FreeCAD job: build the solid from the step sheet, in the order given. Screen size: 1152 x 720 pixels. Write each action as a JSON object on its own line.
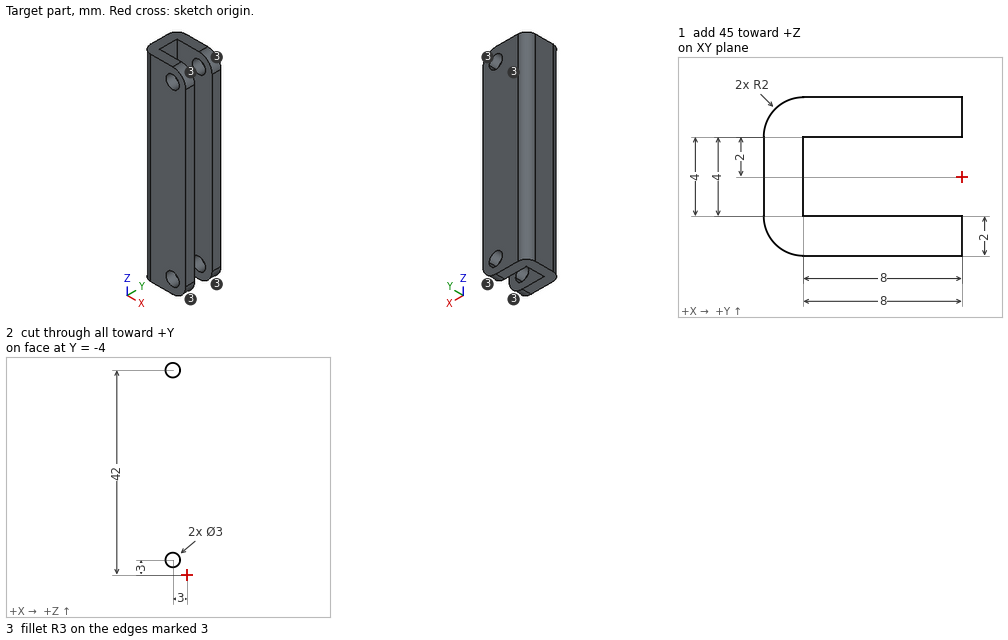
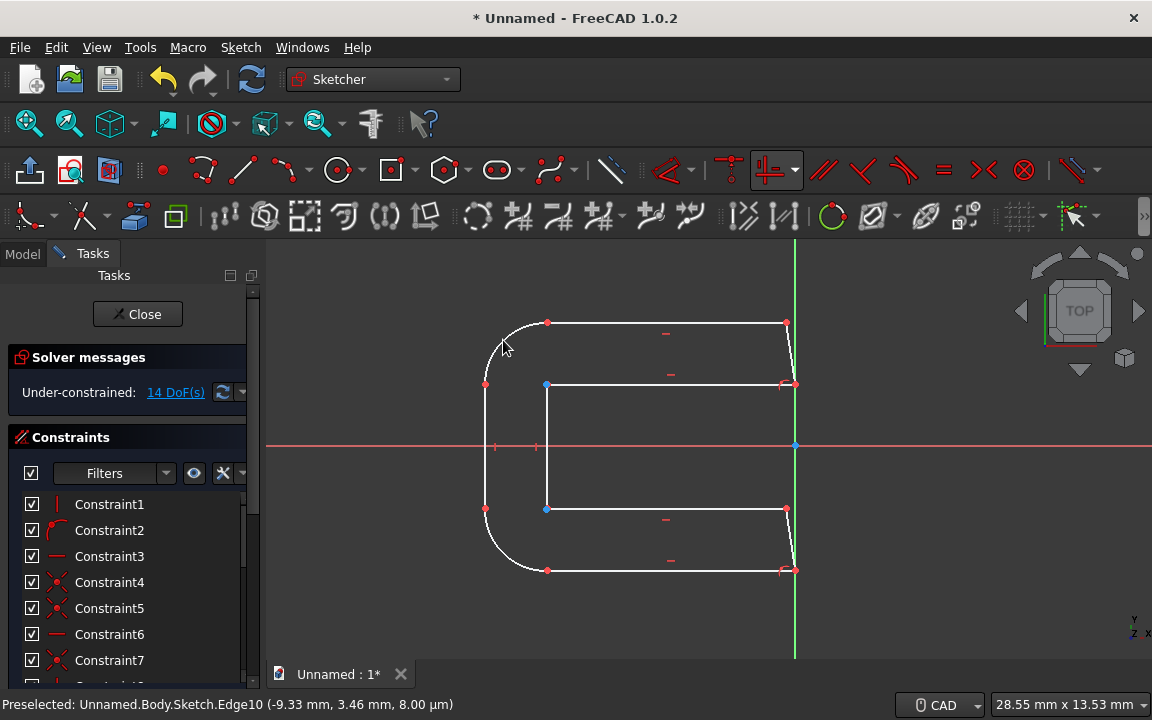
{"action": "left_click", "coordinate": [485, 422]}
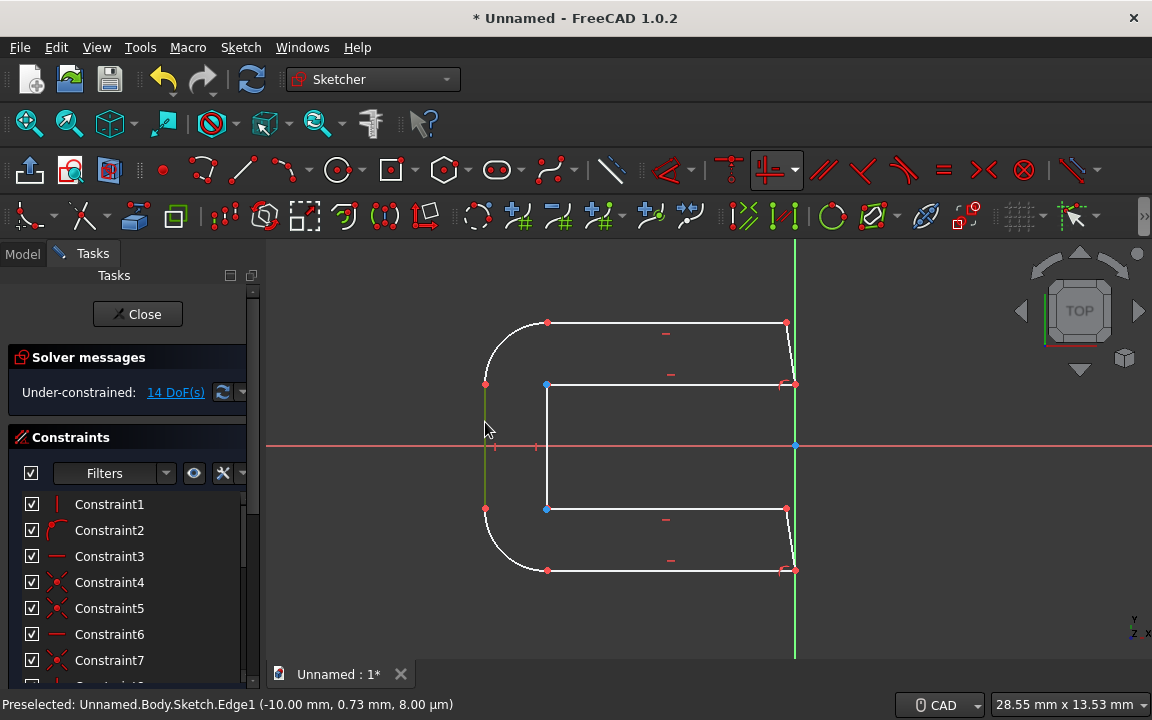
{"action": "left_click", "coordinate": [492, 537]}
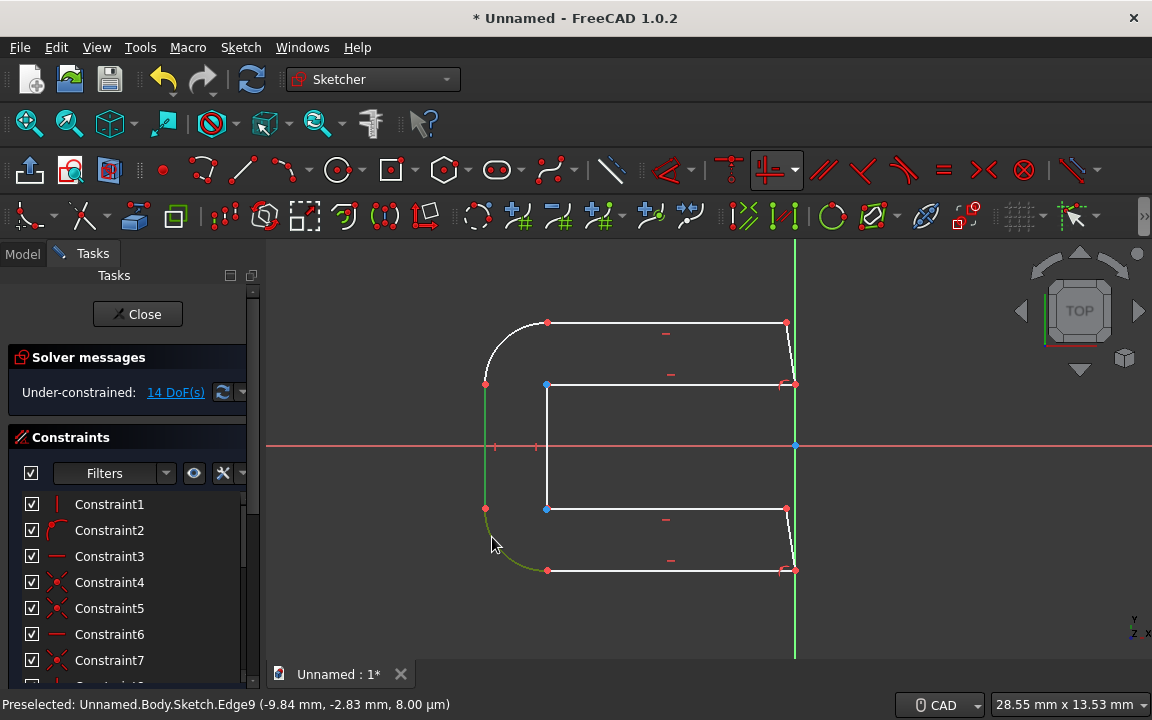
{"action": "left_click", "coordinate": [904, 170]}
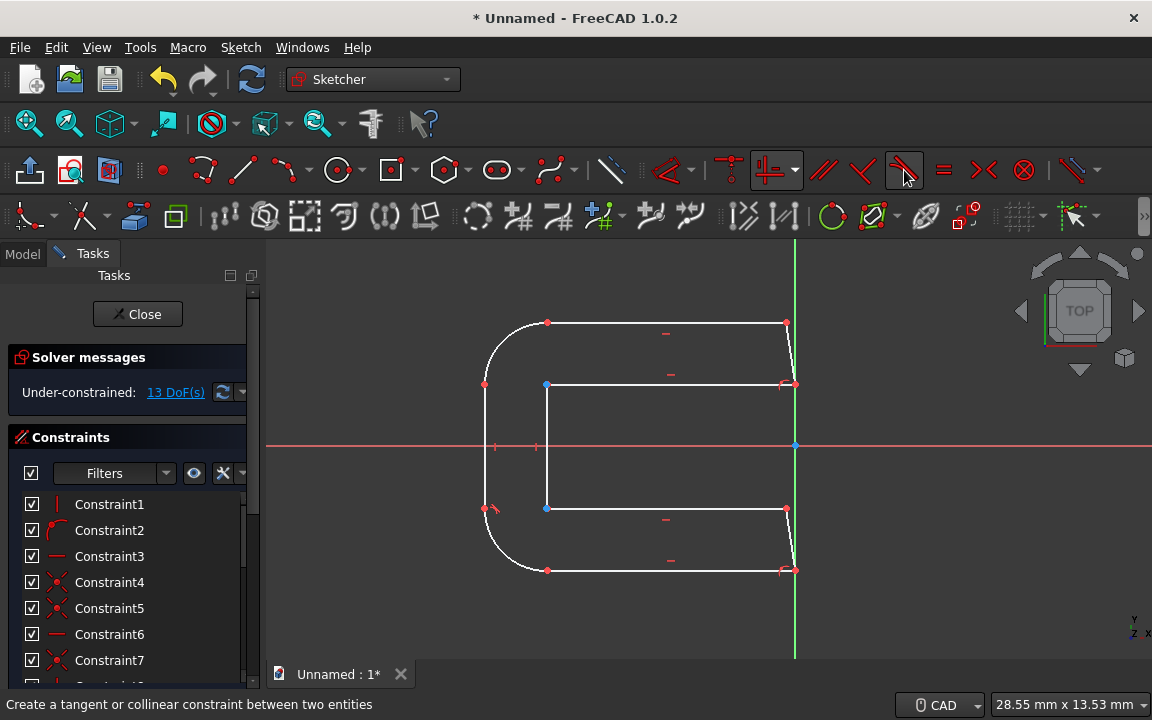
{"action": "left_click", "coordinate": [485, 422]}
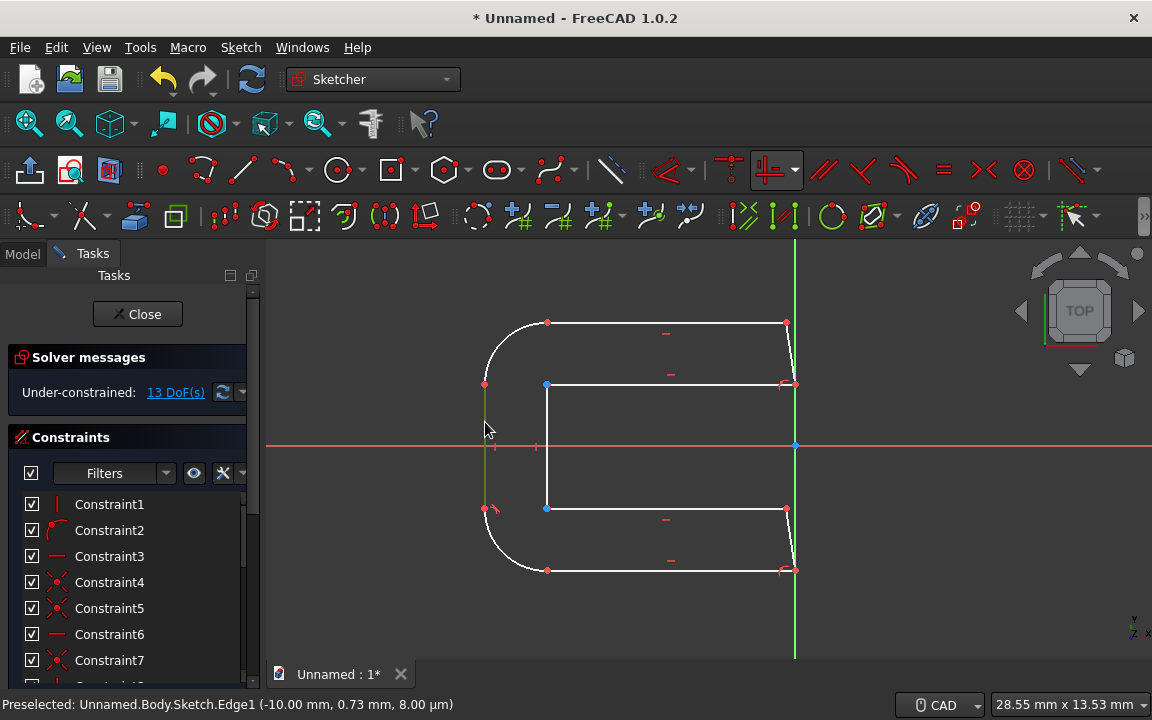
{"action": "left_click", "coordinate": [519, 330]}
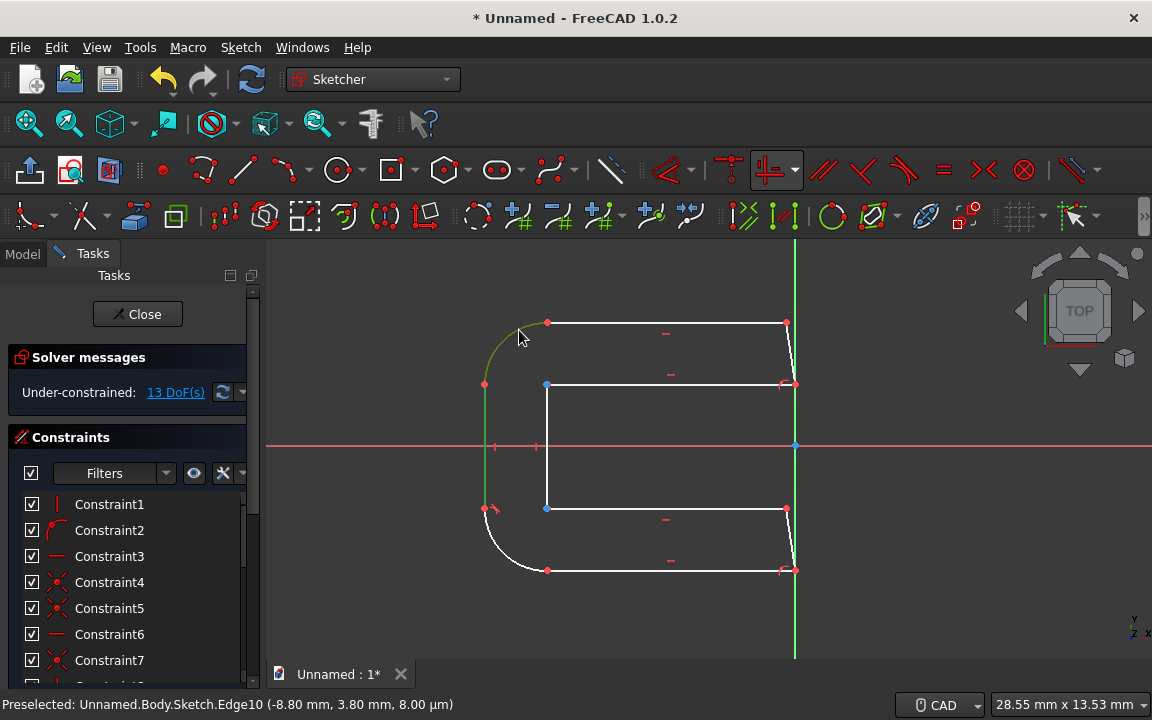
{"action": "left_click", "coordinate": [904, 170]}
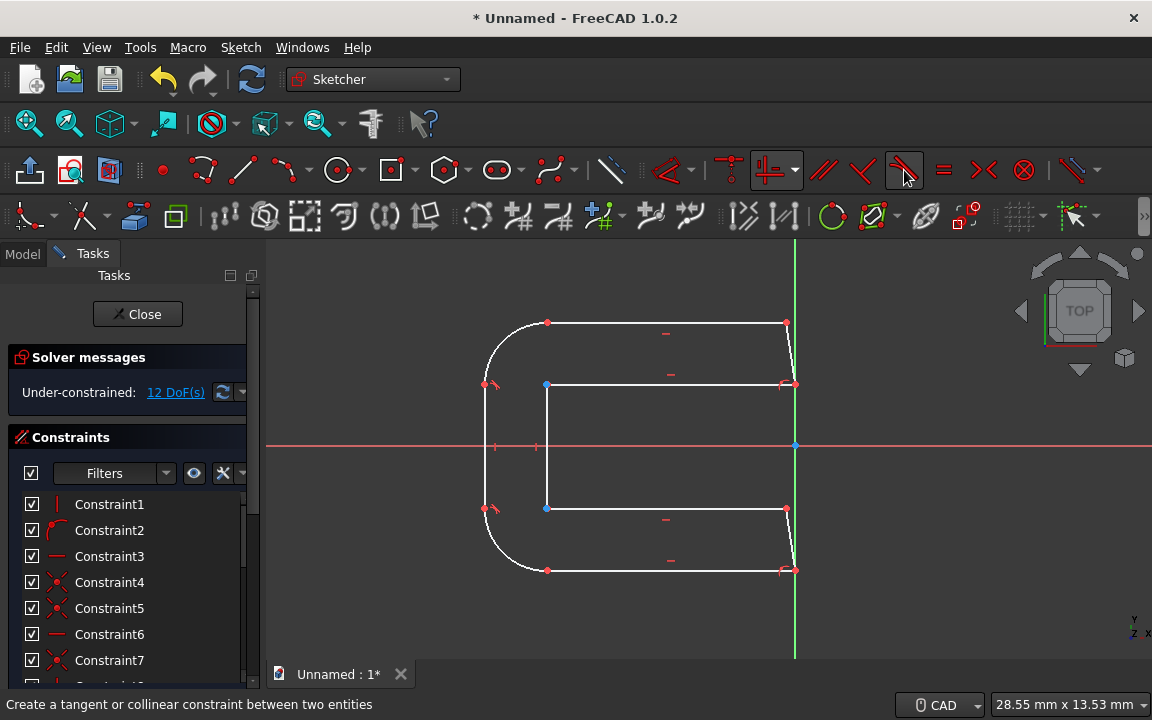
{"action": "left_click", "coordinate": [622, 571]}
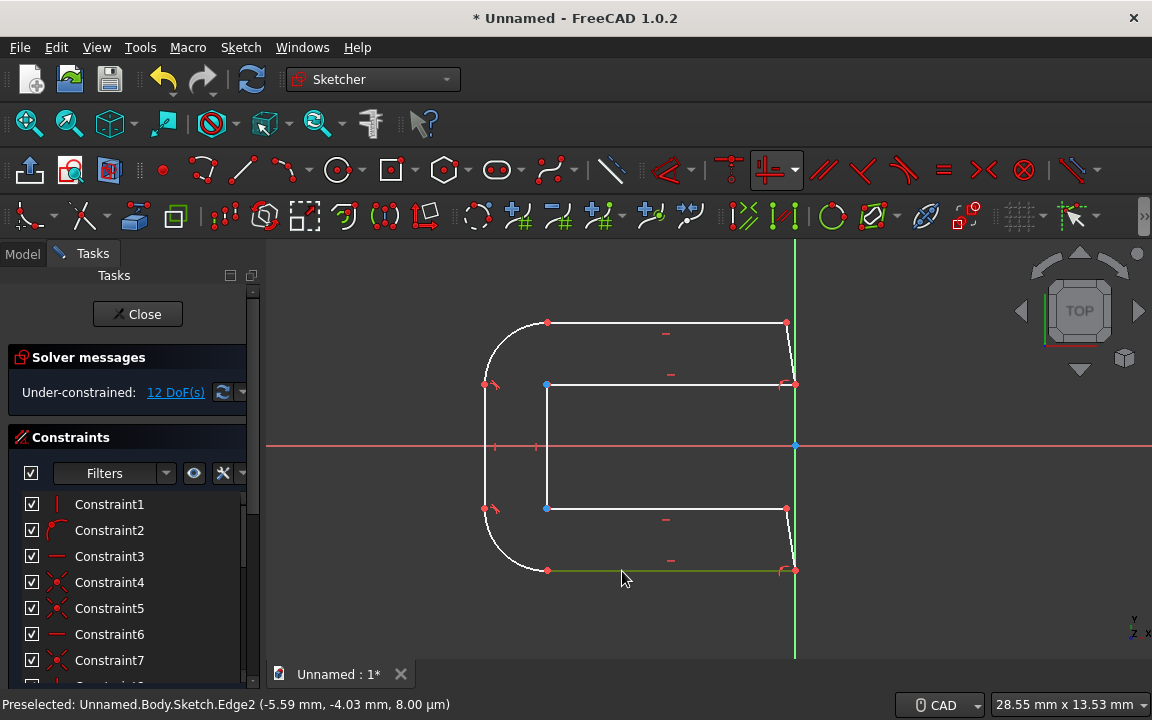
{"action": "left_click", "coordinate": [492, 537]}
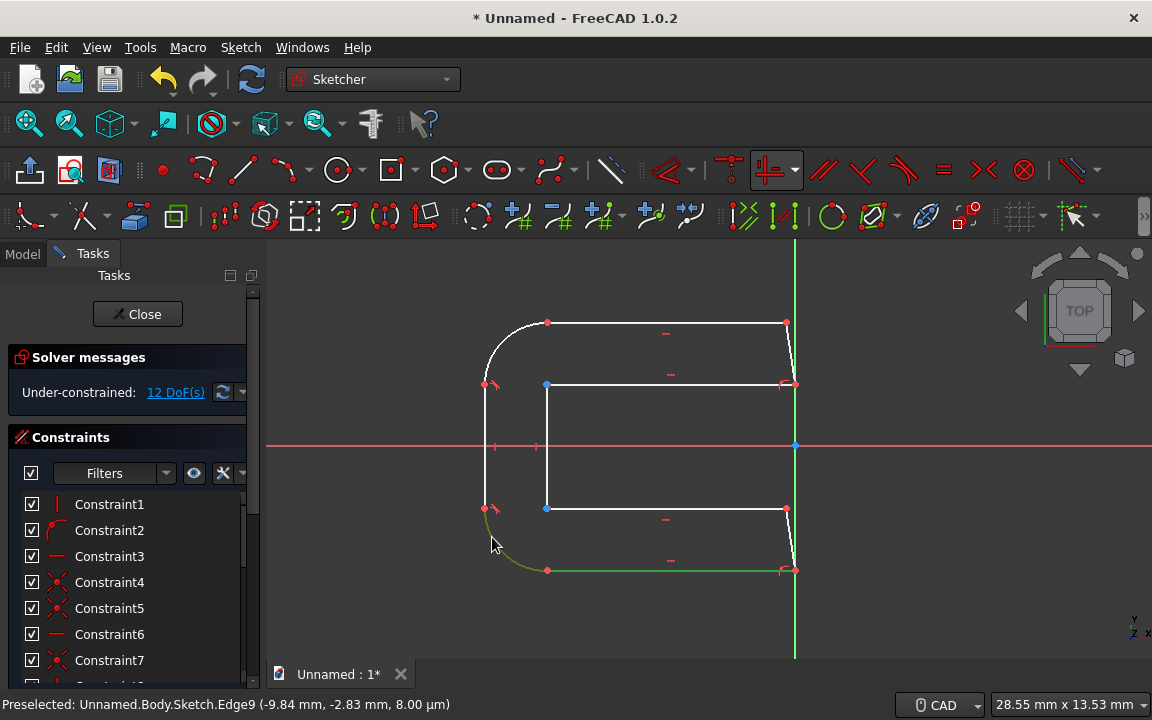
{"action": "left_click", "coordinate": [904, 170]}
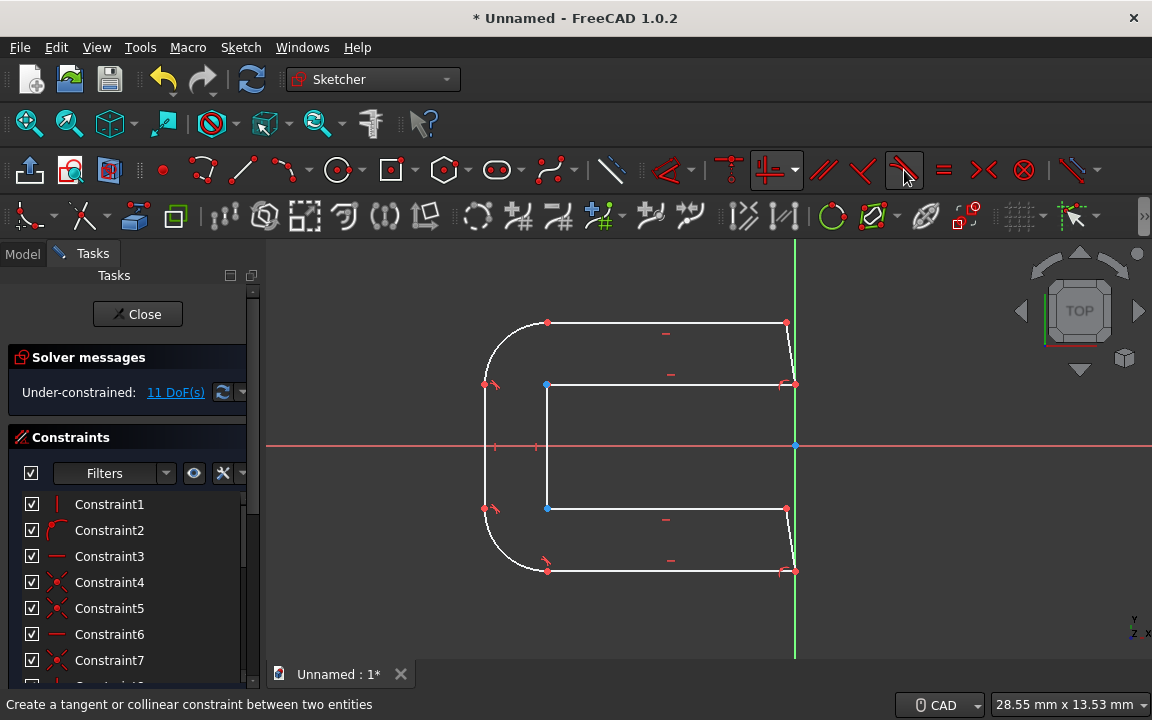
{"action": "left_click", "coordinate": [714, 323]}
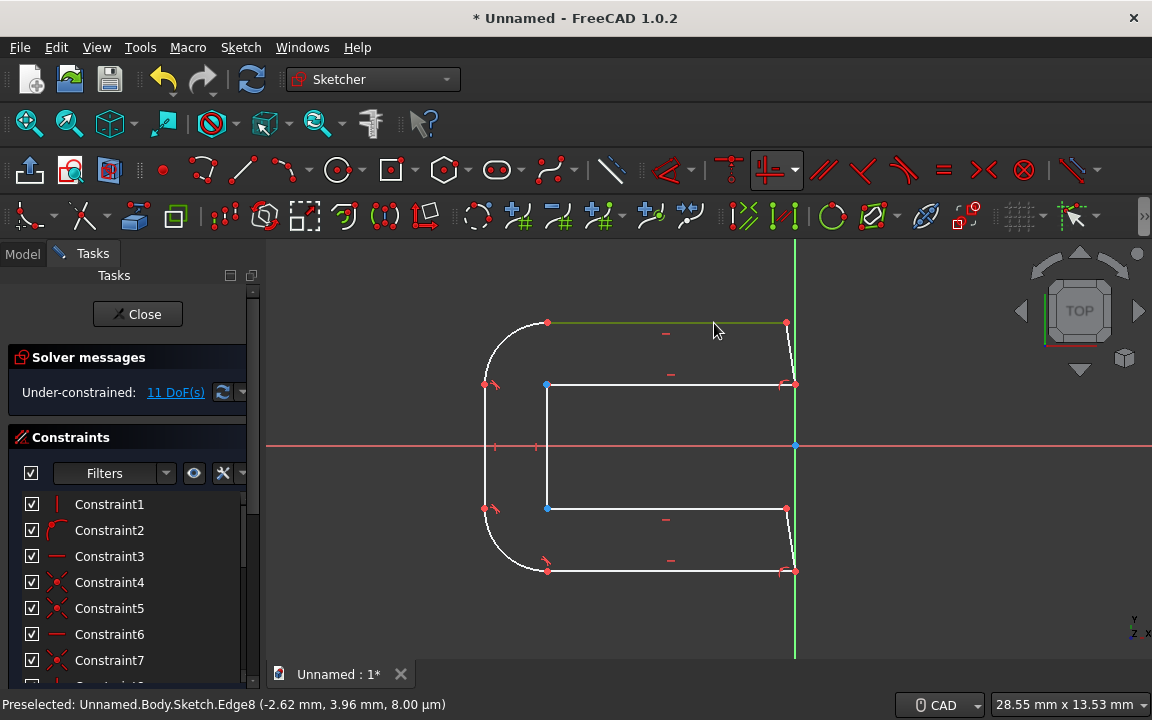
{"action": "left_click", "coordinate": [519, 330]}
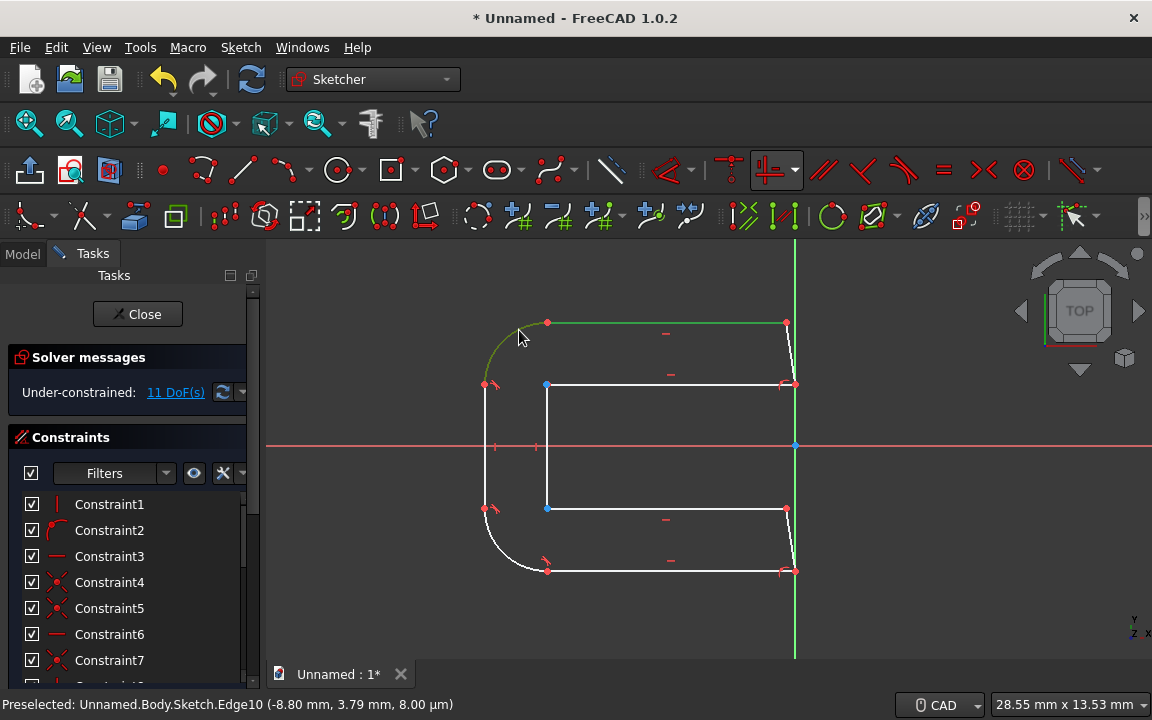
{"action": "left_click", "coordinate": [904, 170]}